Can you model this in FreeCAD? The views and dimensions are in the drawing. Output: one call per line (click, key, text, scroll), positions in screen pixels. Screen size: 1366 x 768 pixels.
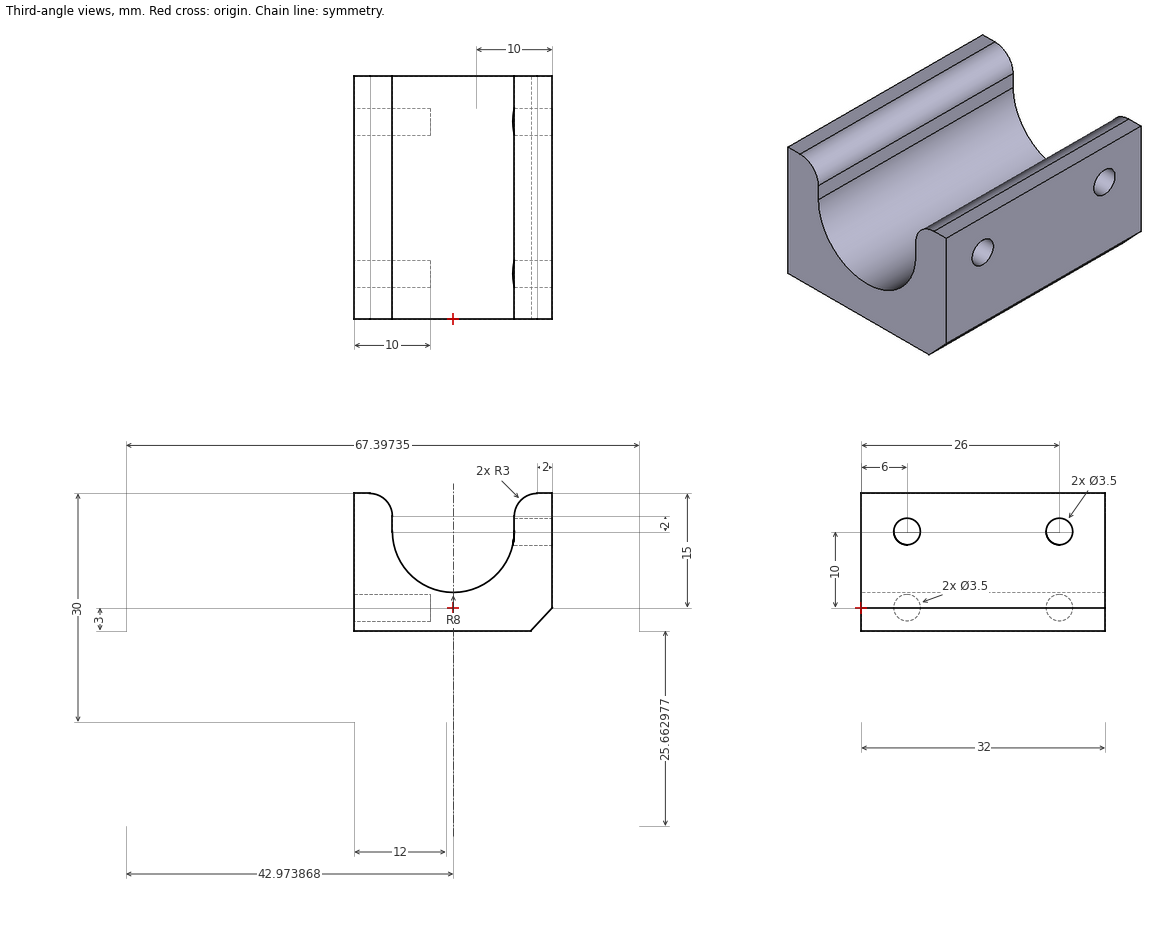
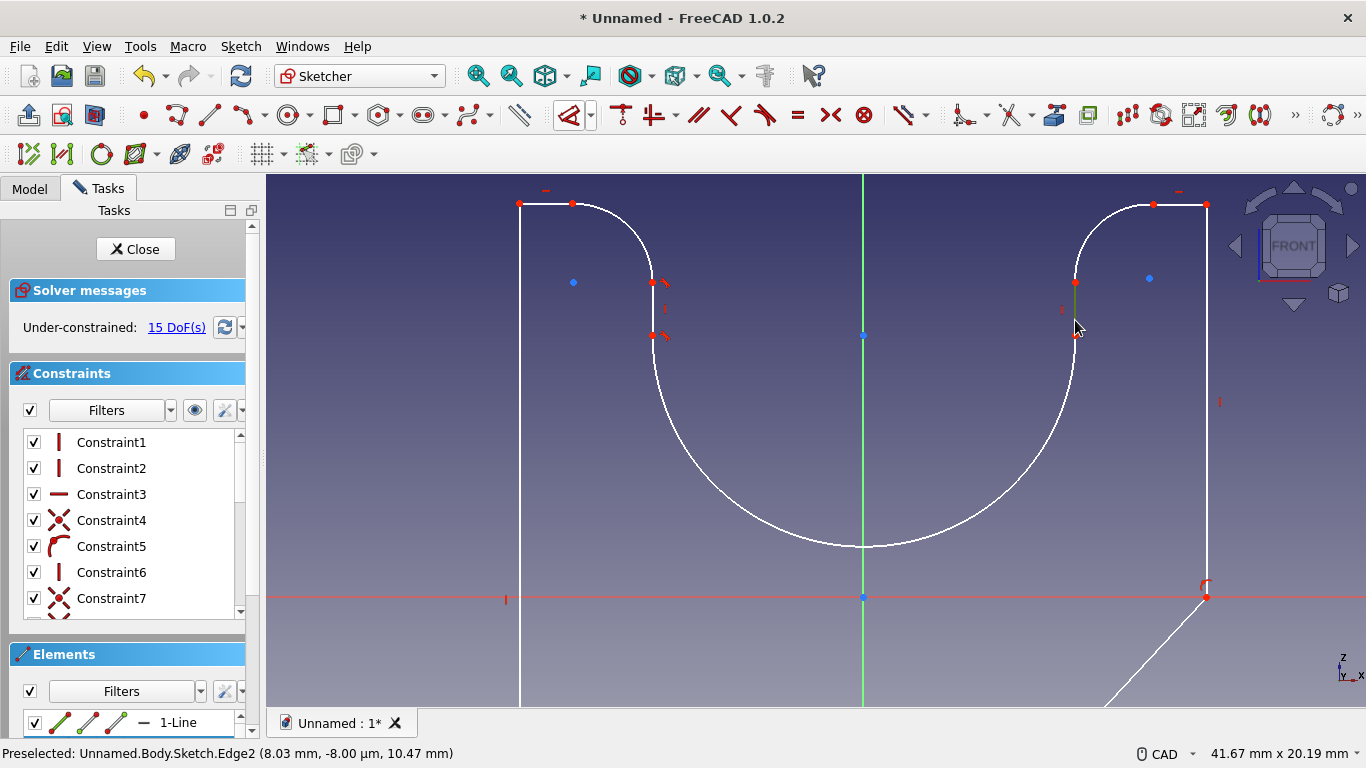
click(740, 506)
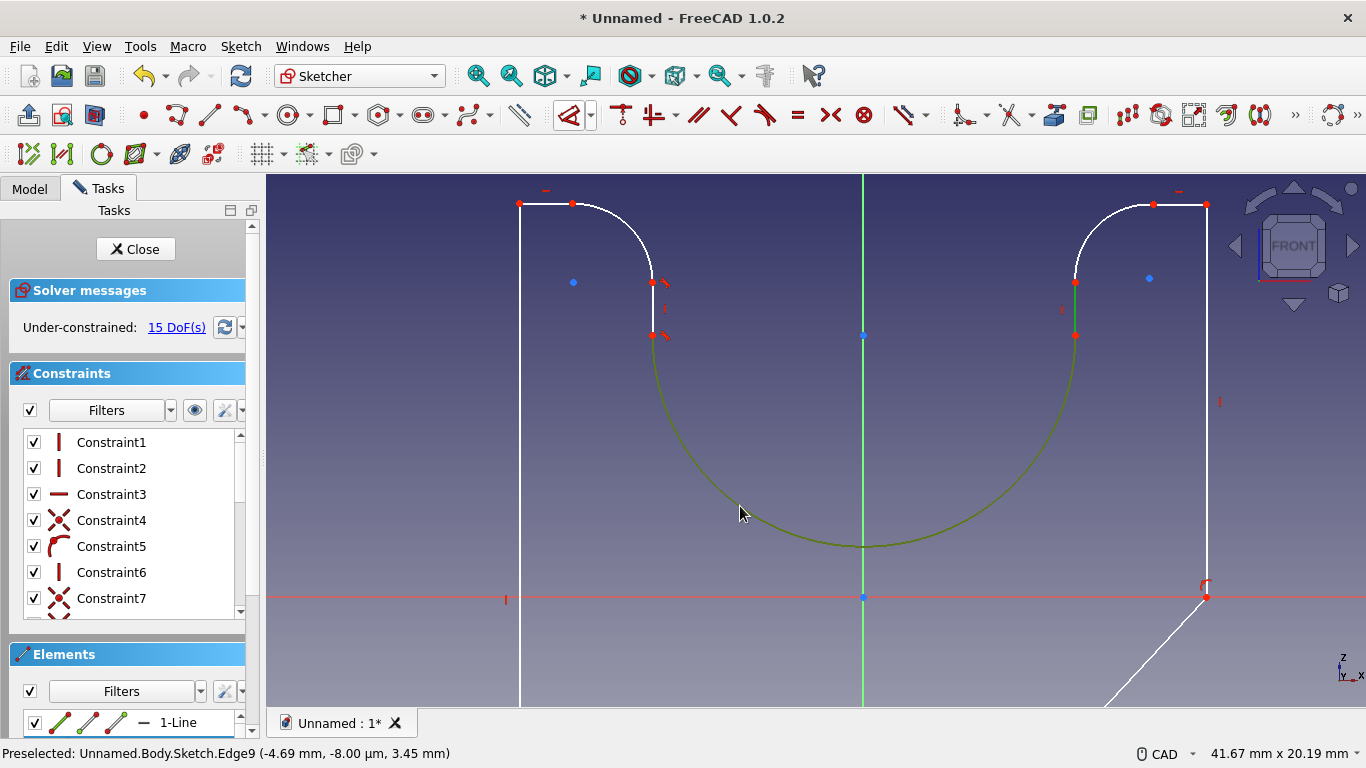
click(765, 116)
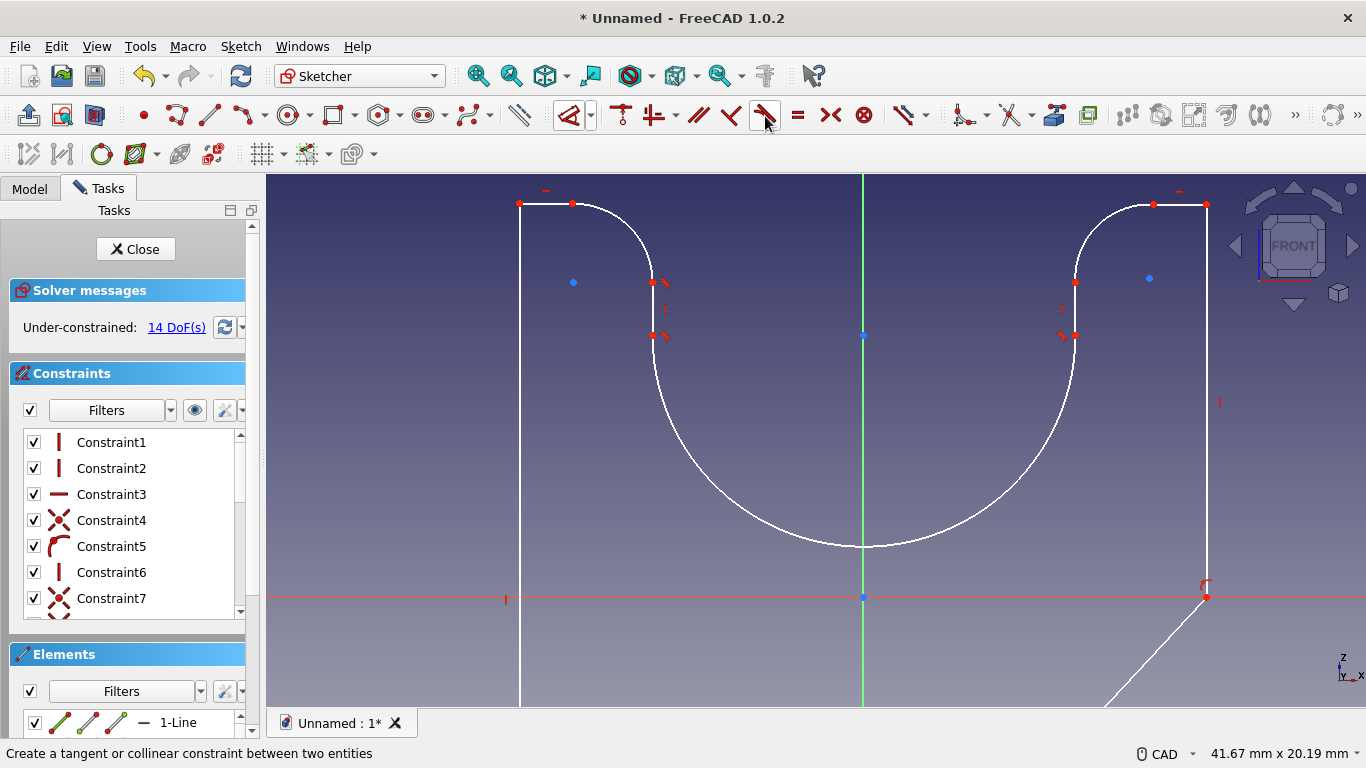
click(1075, 320)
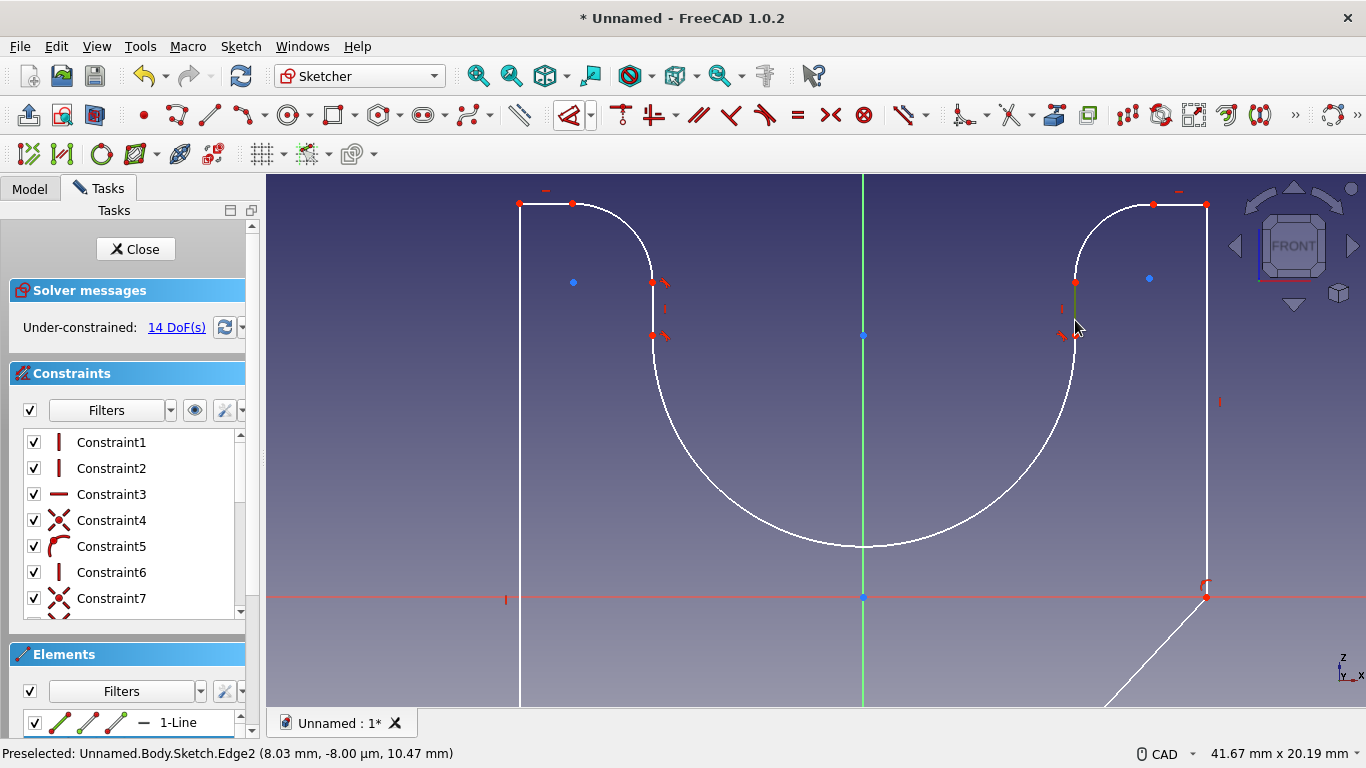
click(1117, 212)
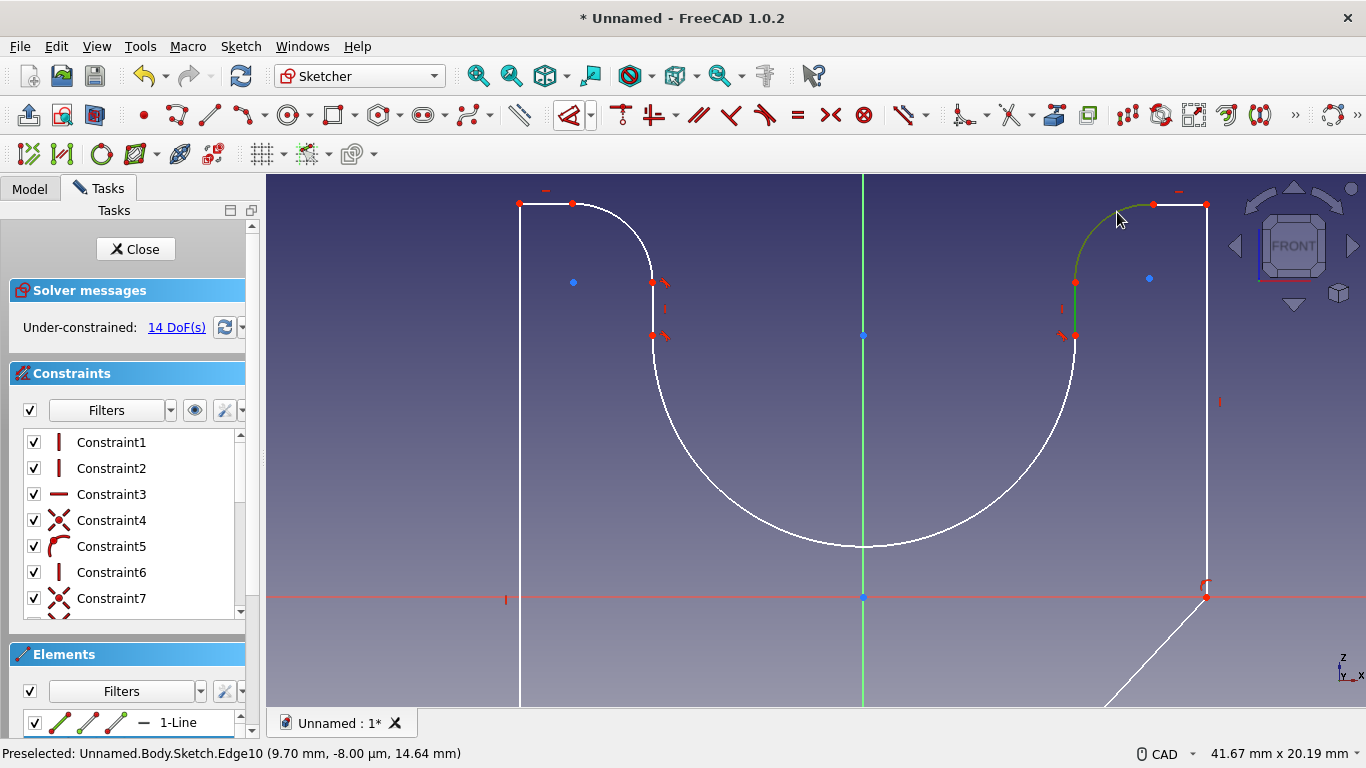
click(765, 116)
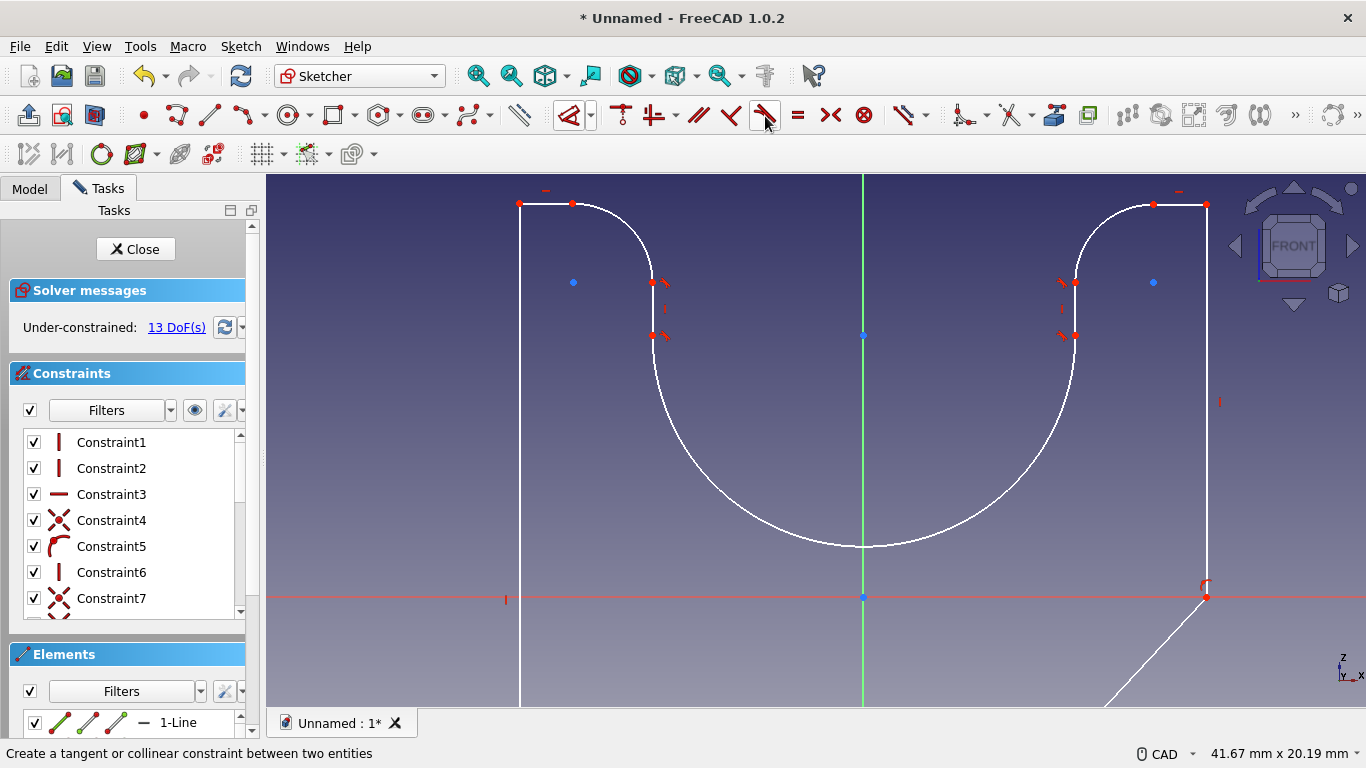
click(1169, 205)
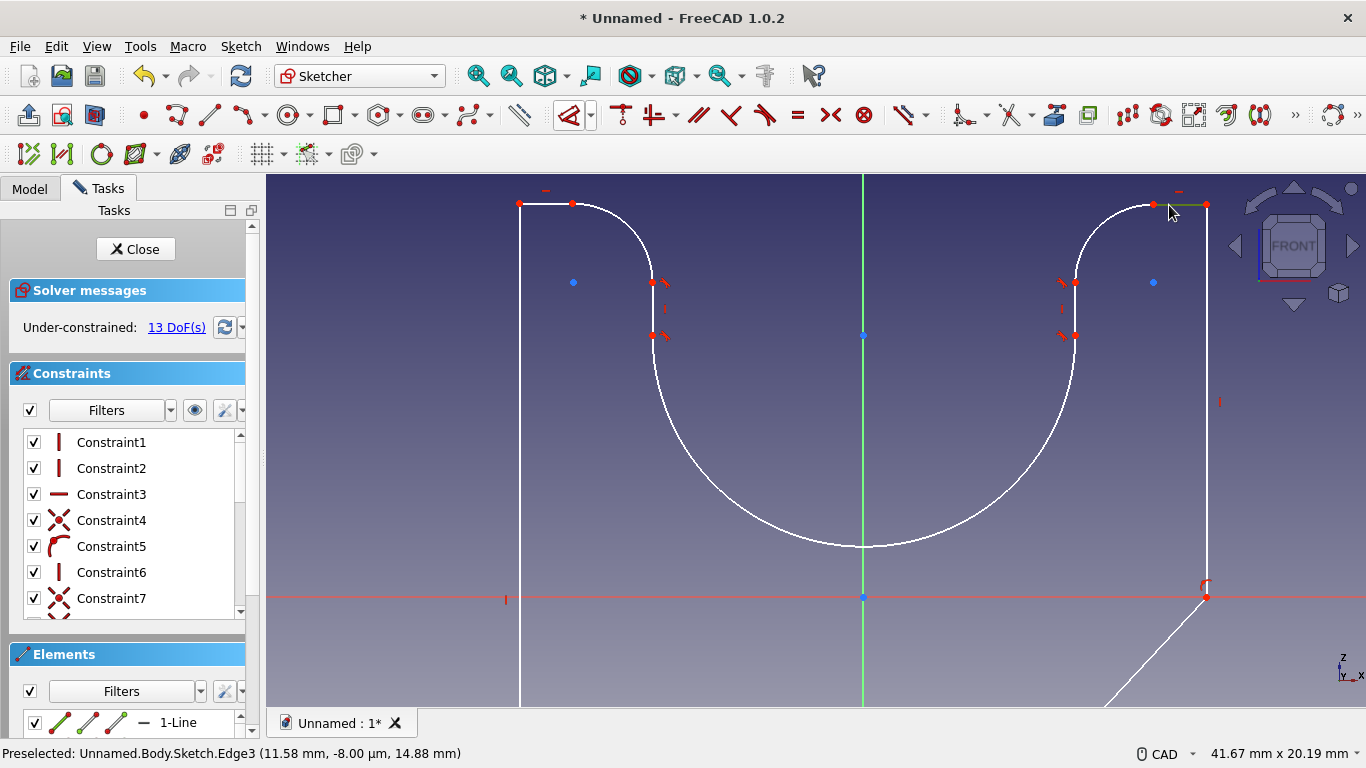
click(1118, 213)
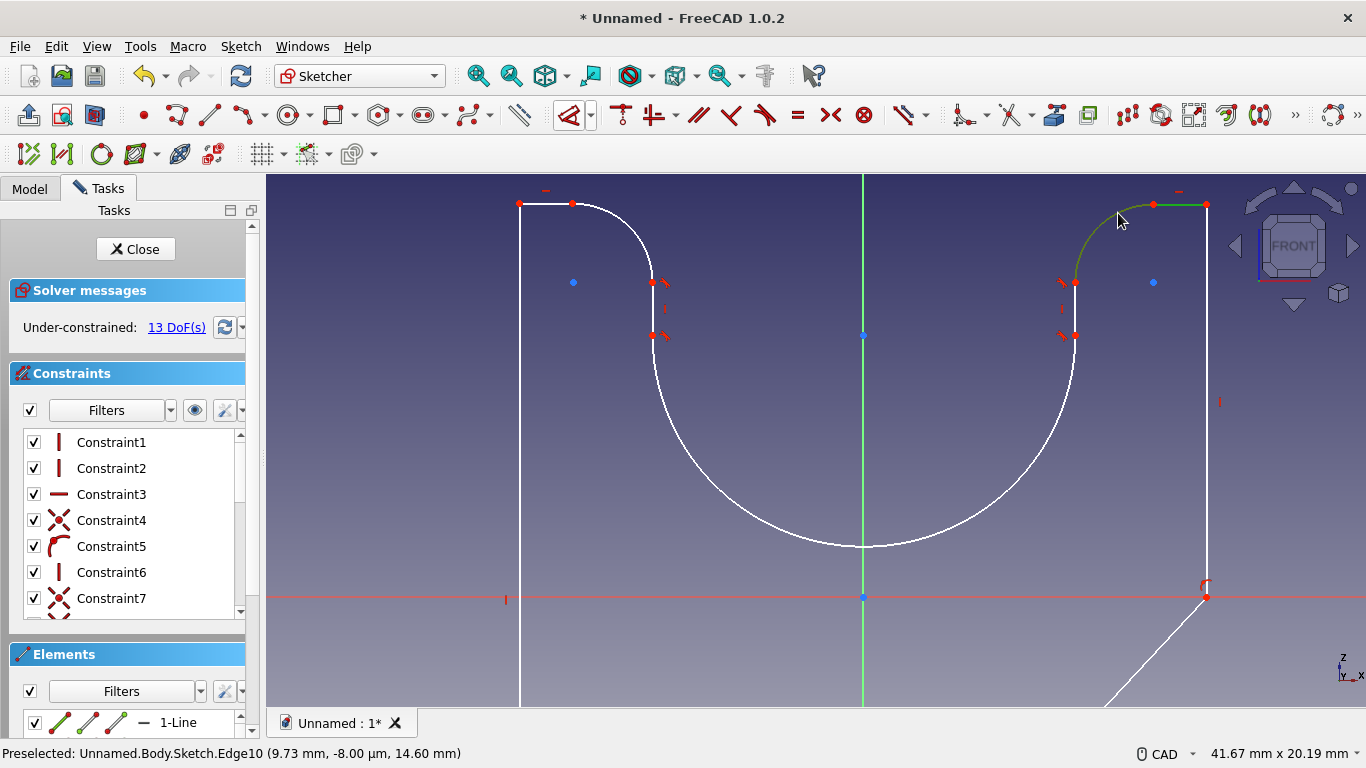
click(765, 116)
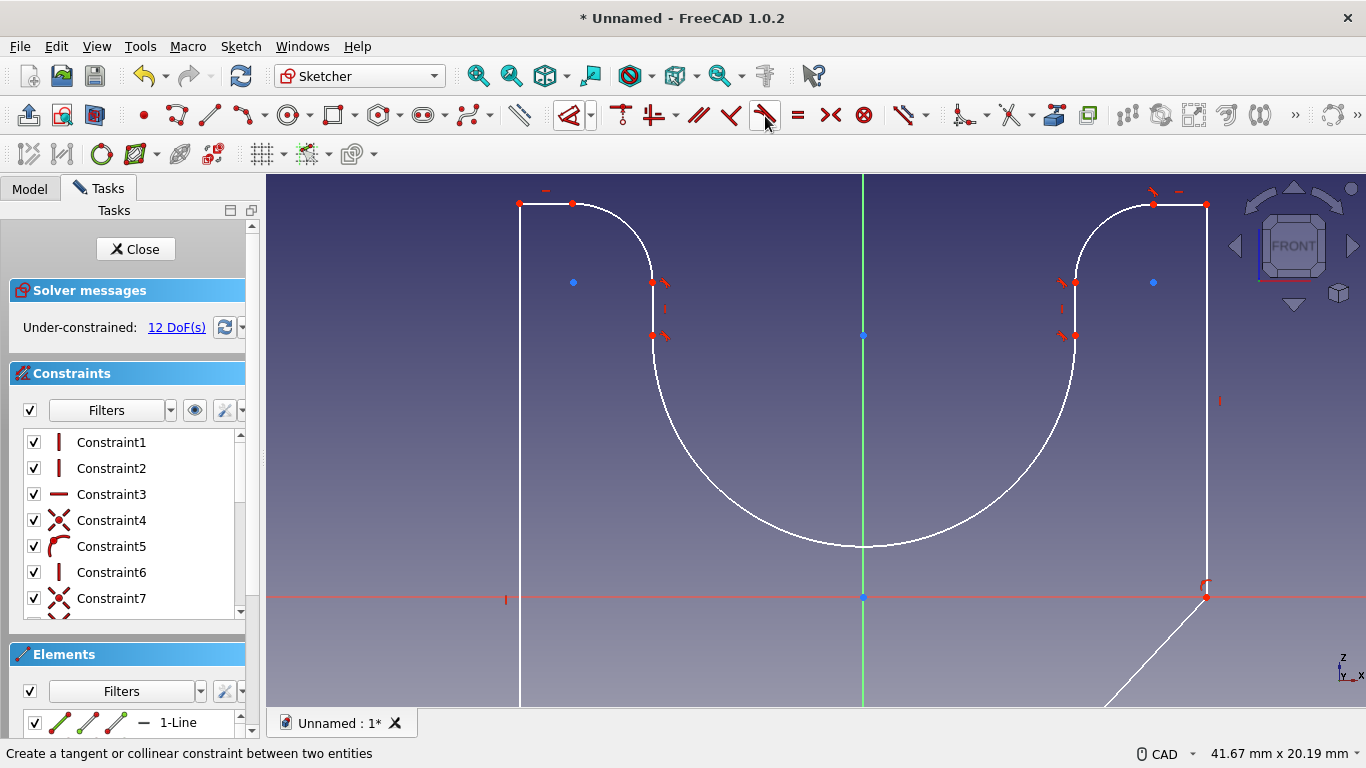
click(536, 204)